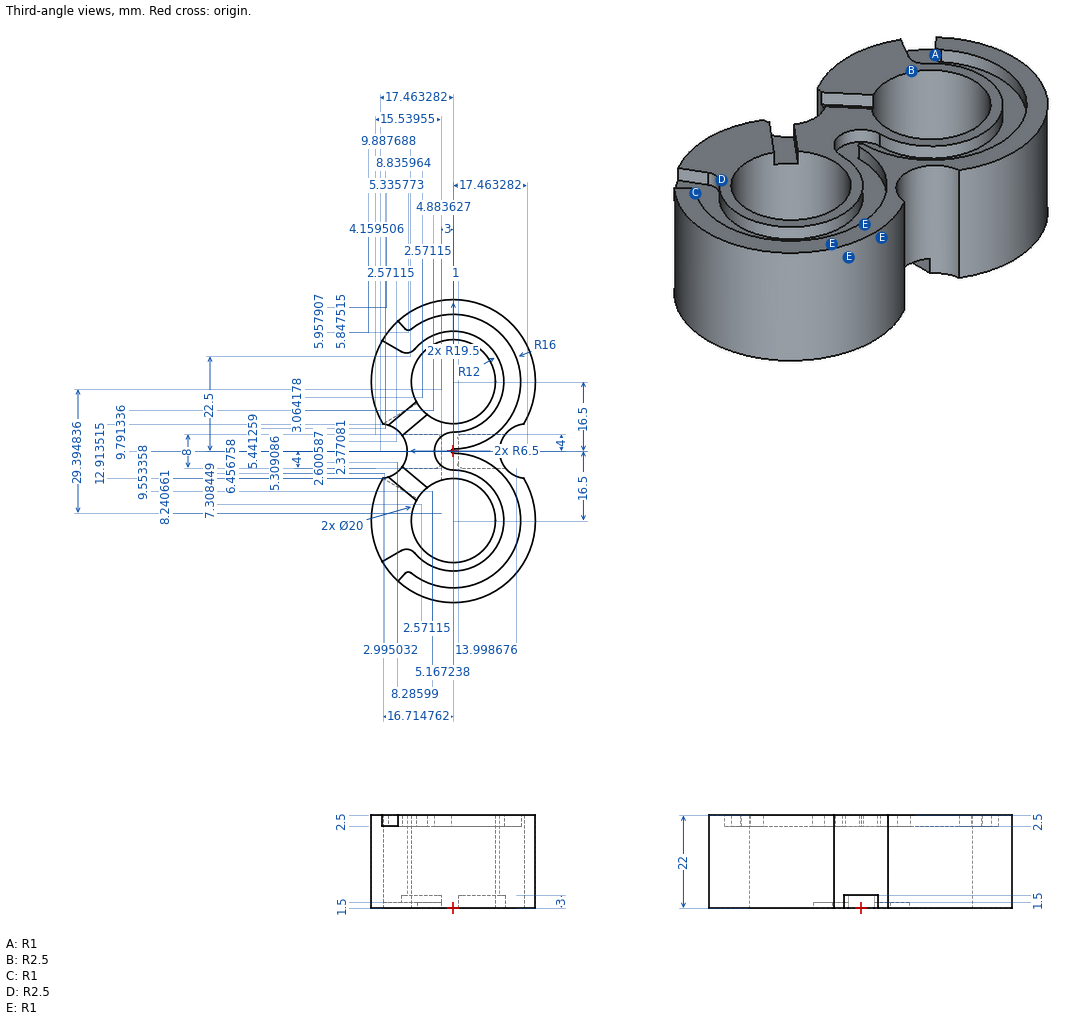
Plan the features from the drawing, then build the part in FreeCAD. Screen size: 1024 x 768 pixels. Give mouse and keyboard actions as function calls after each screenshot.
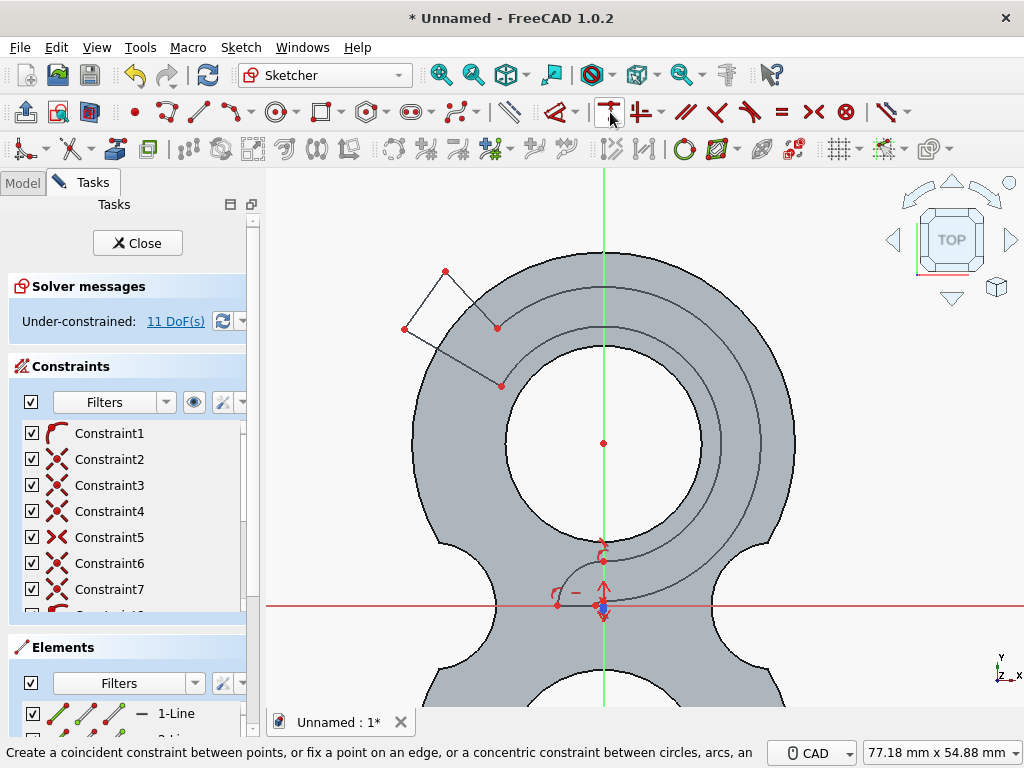
scroll(604, 607, up, 10)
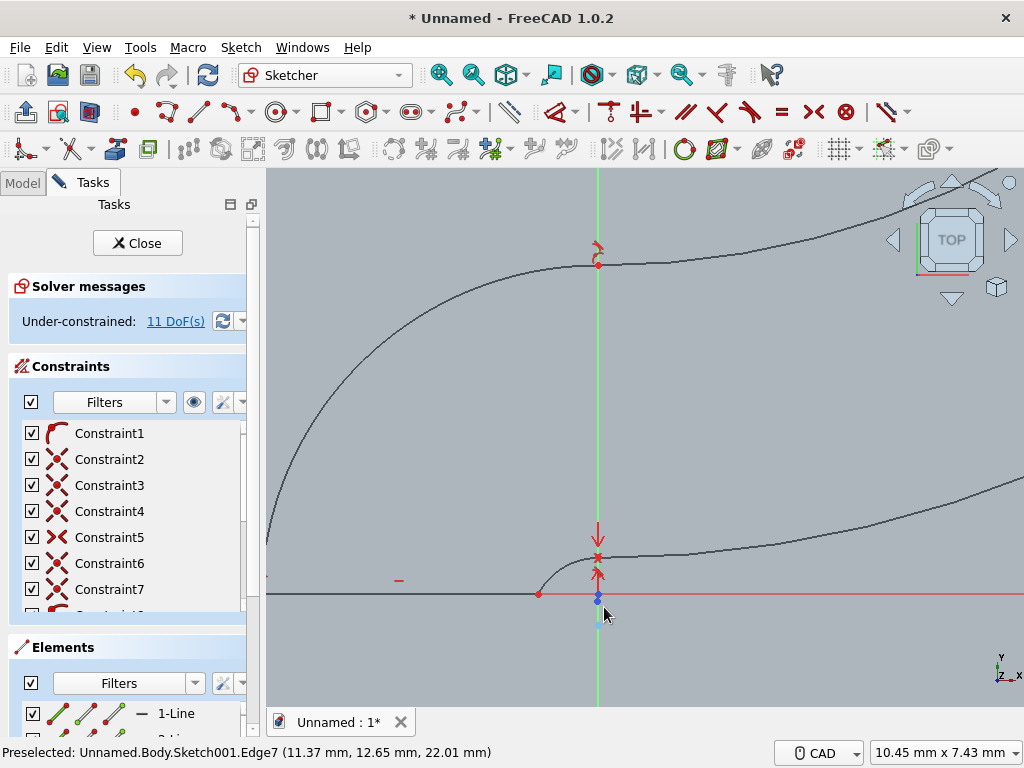
drag(588, 584, 608, 612)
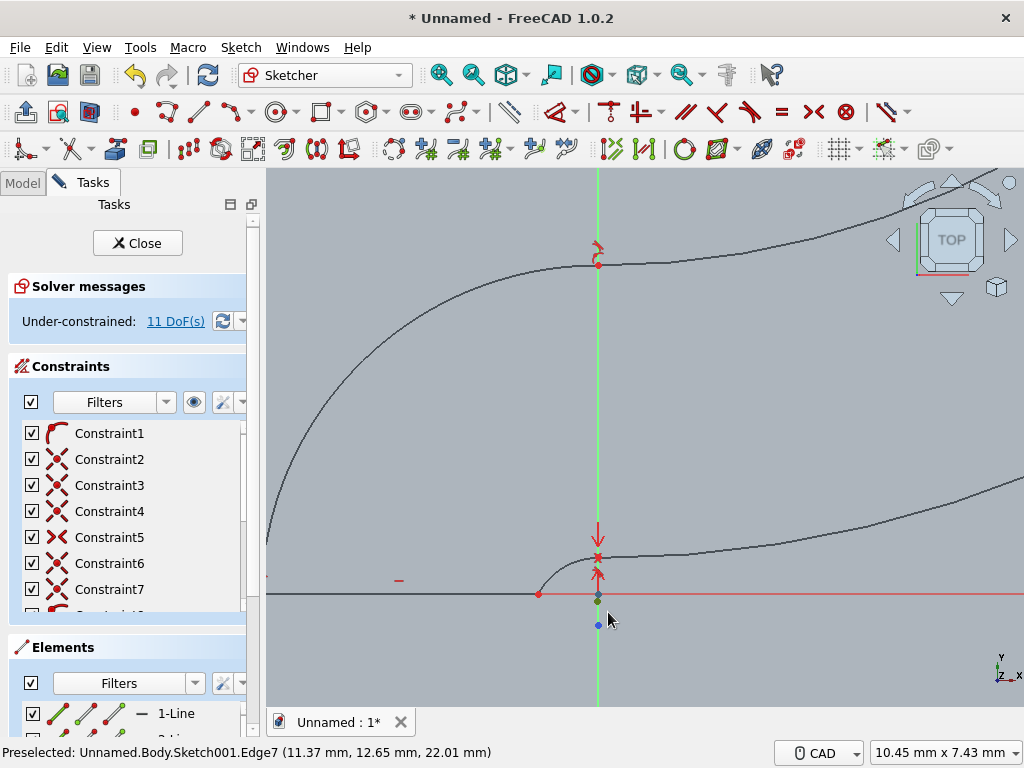
key(c)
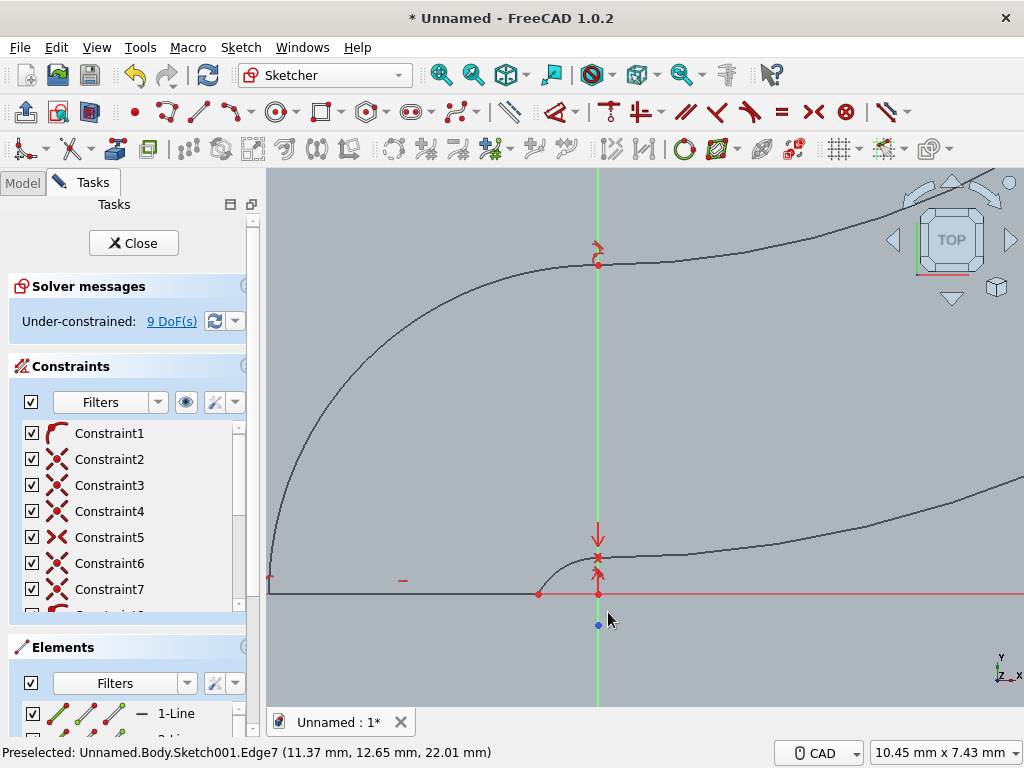
scroll(604, 607, down, 10)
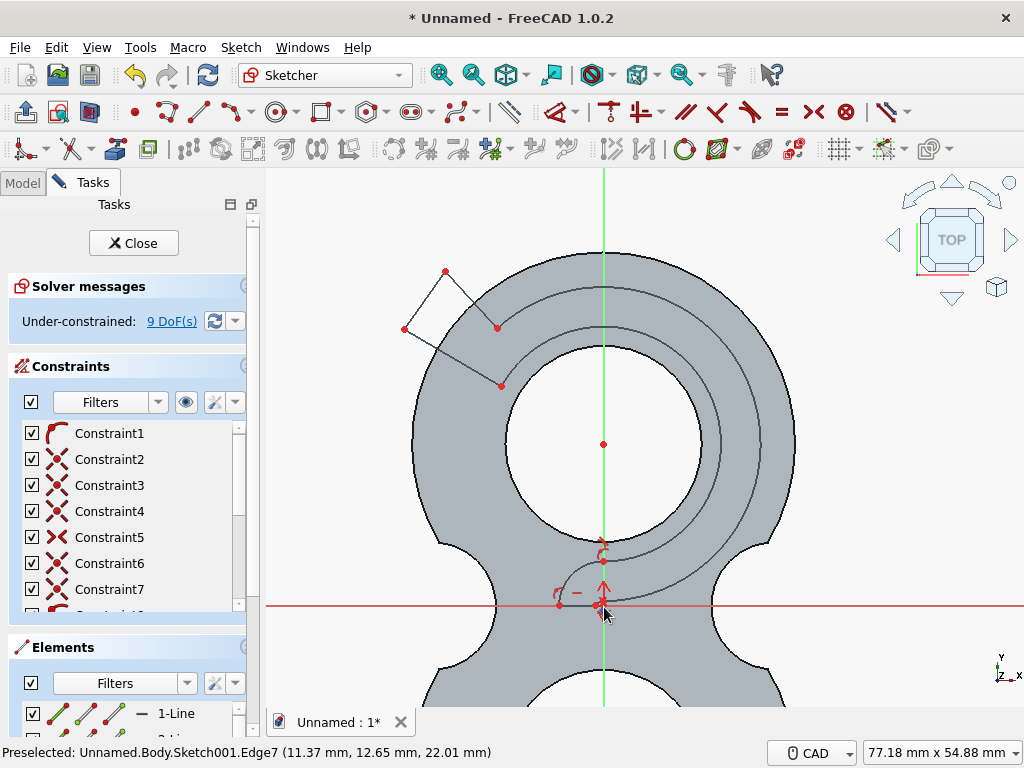
scroll(604, 610, up, 2)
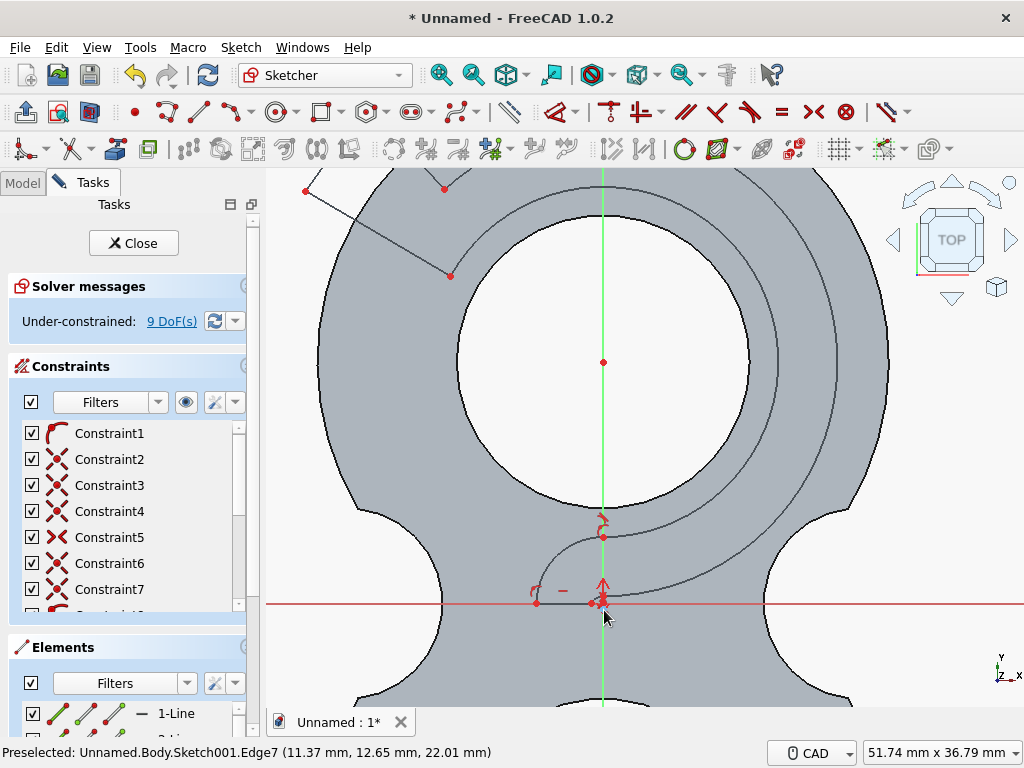
click(603, 610)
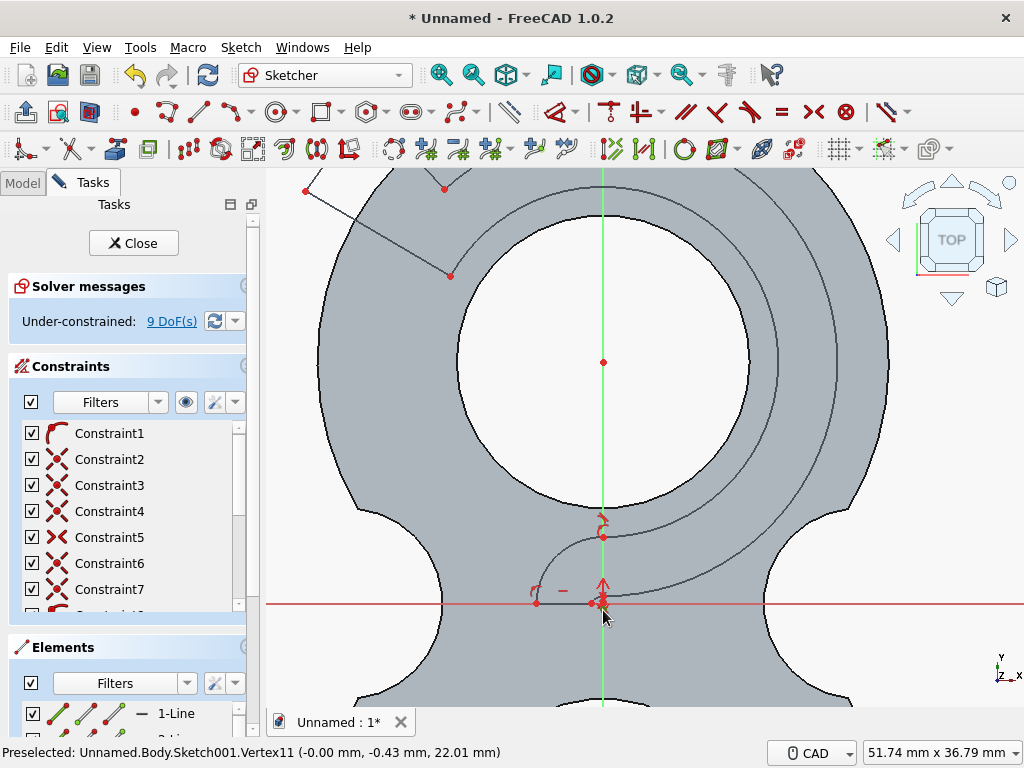
click(334, 604)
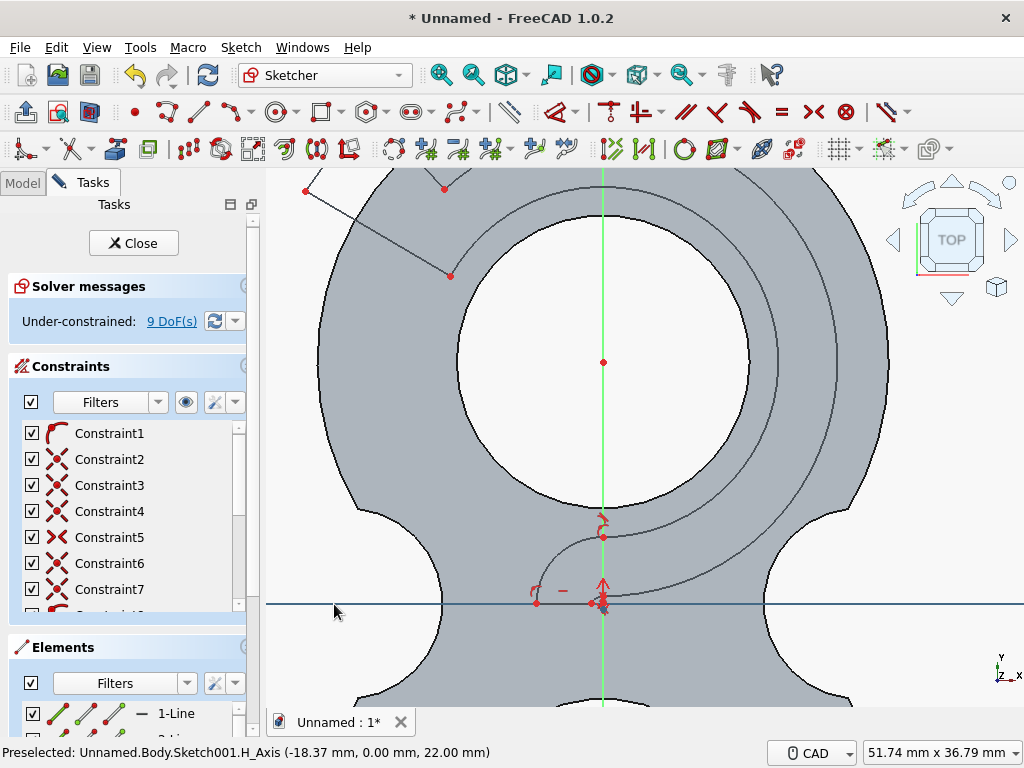
key(c)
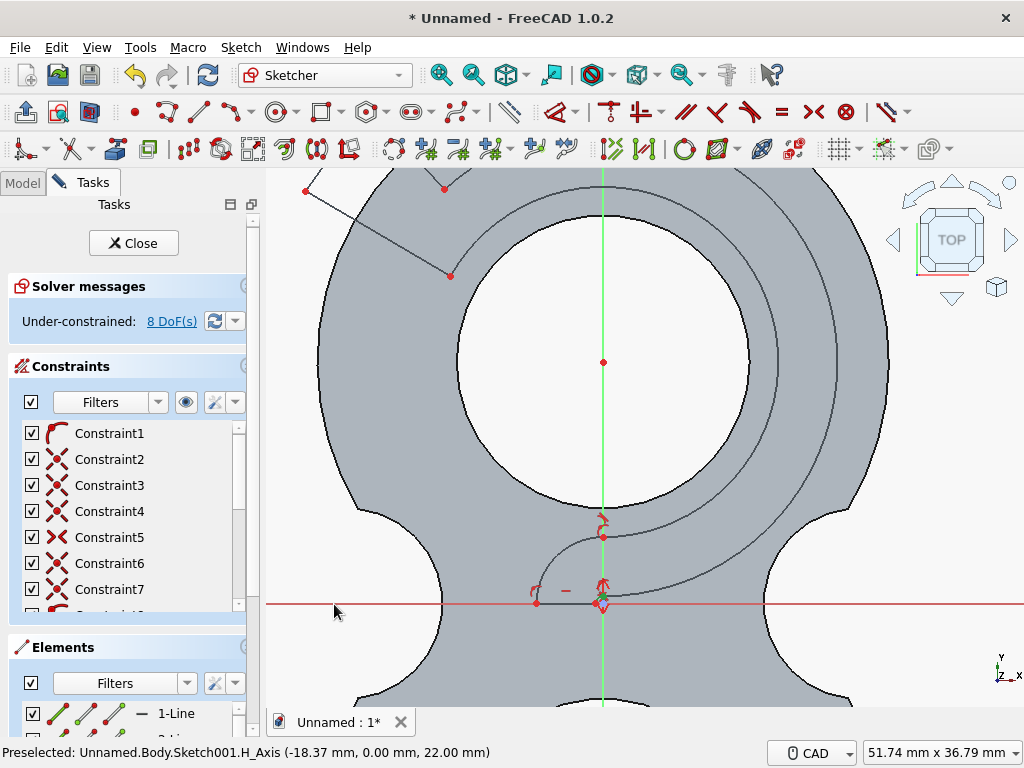
click(818, 454)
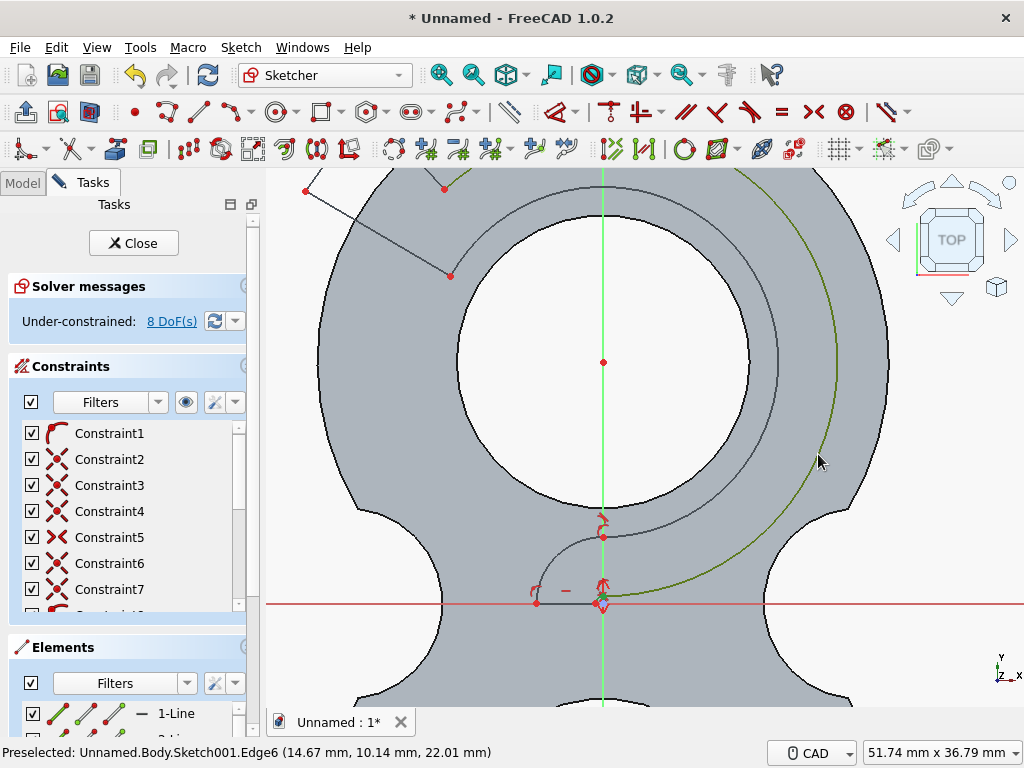
key(k)
key(r)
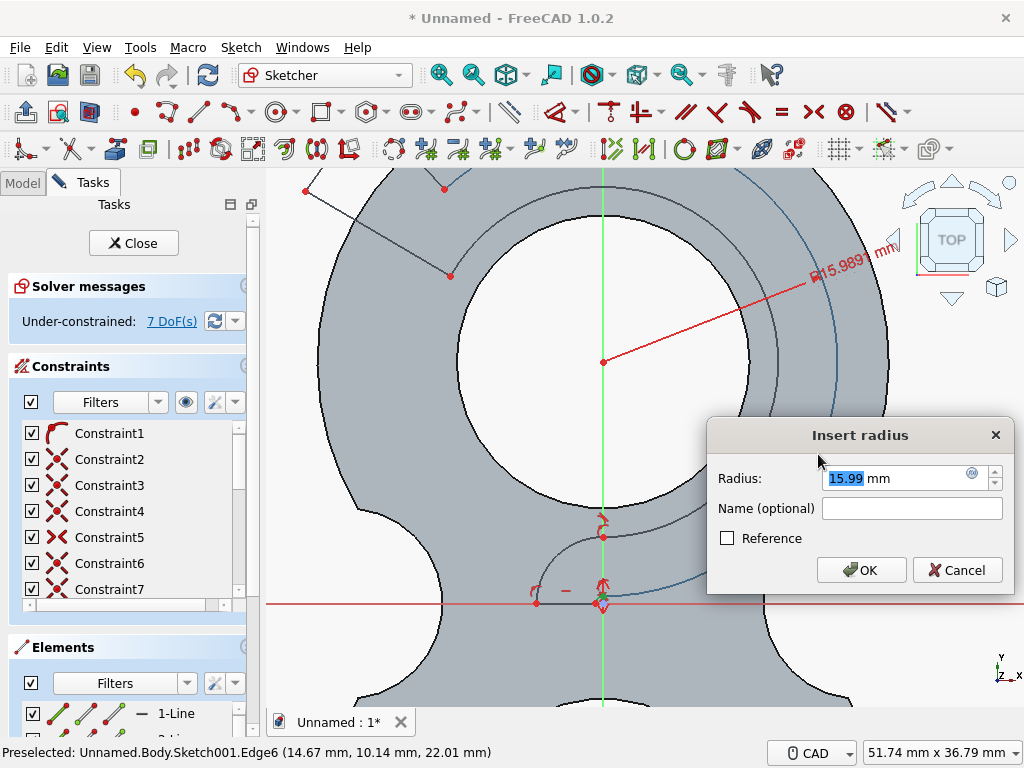
text(16)
key(Return)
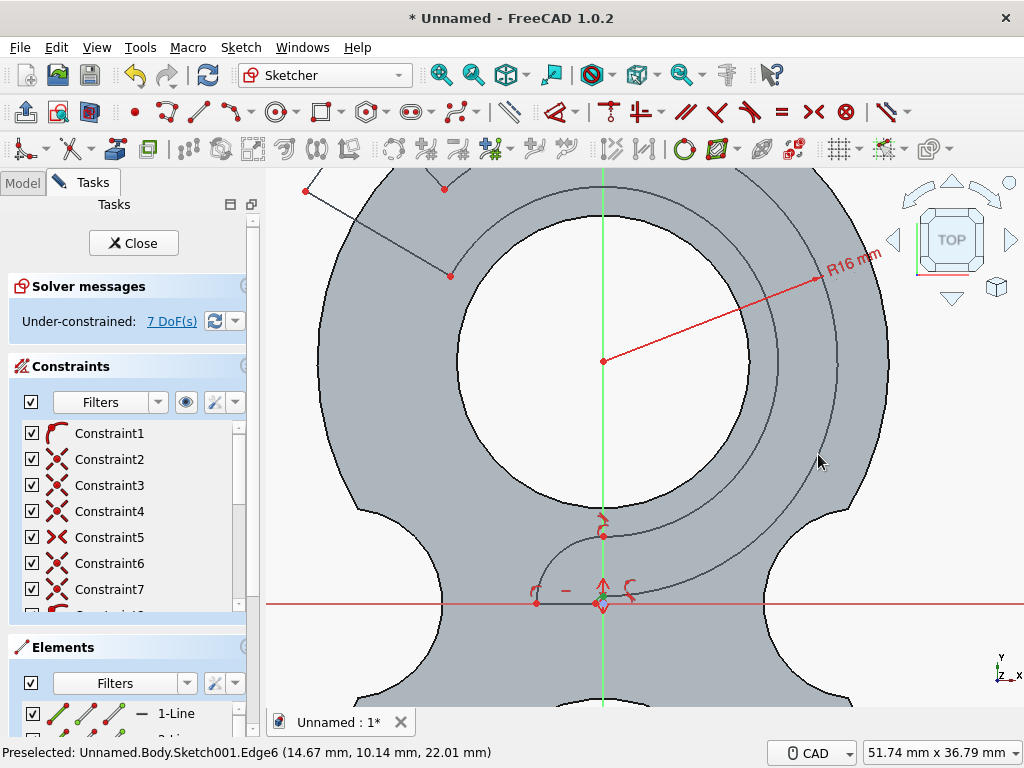
click(770, 415)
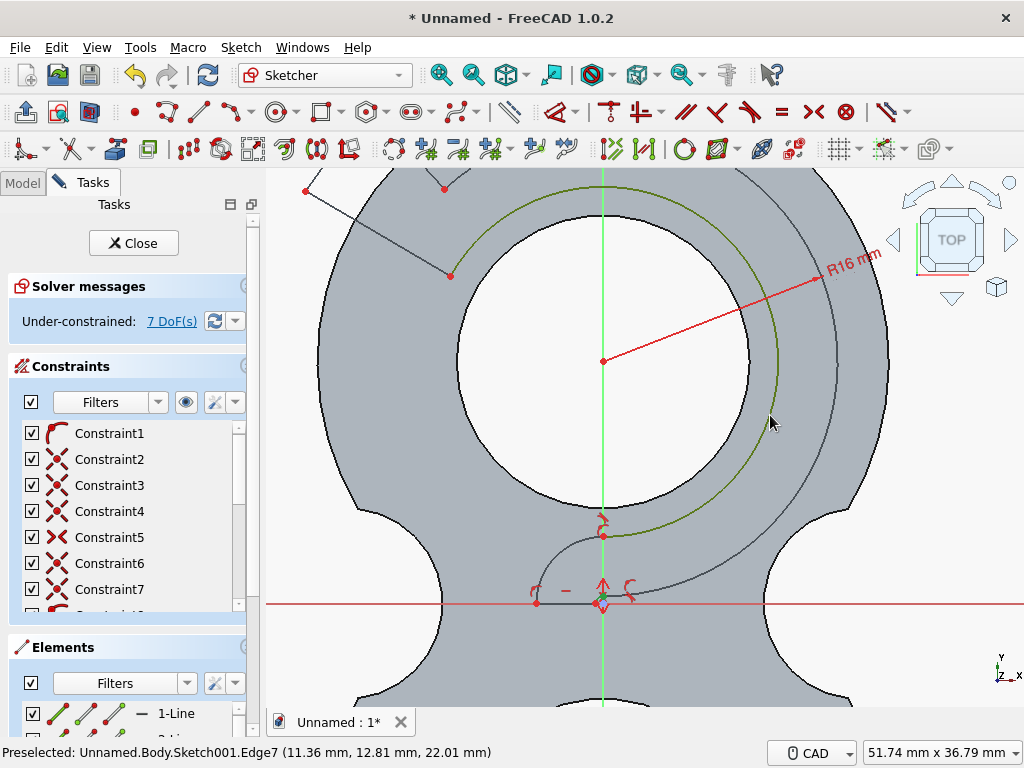
key(k)
key(r)